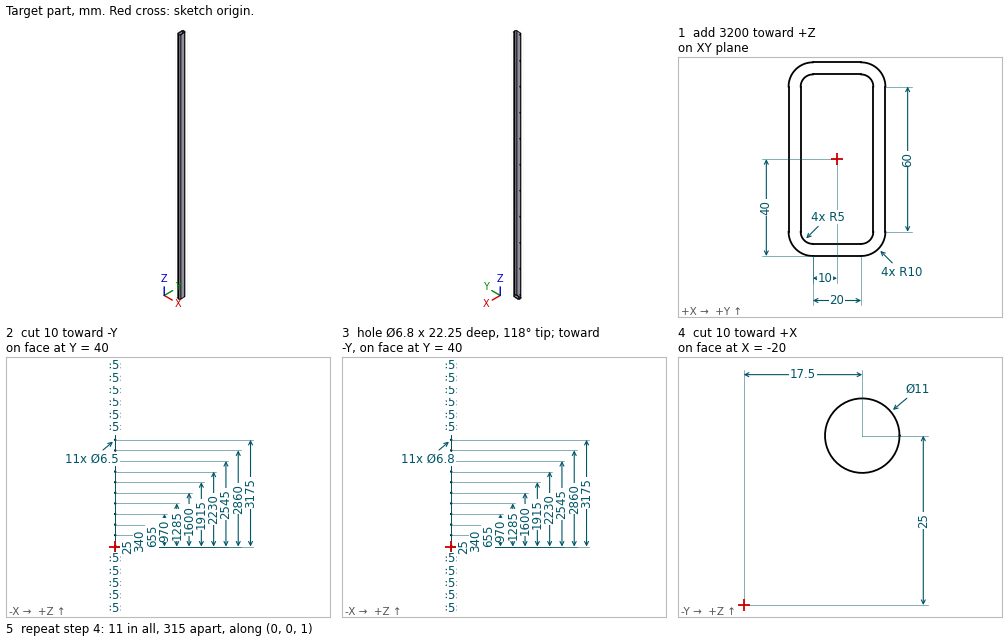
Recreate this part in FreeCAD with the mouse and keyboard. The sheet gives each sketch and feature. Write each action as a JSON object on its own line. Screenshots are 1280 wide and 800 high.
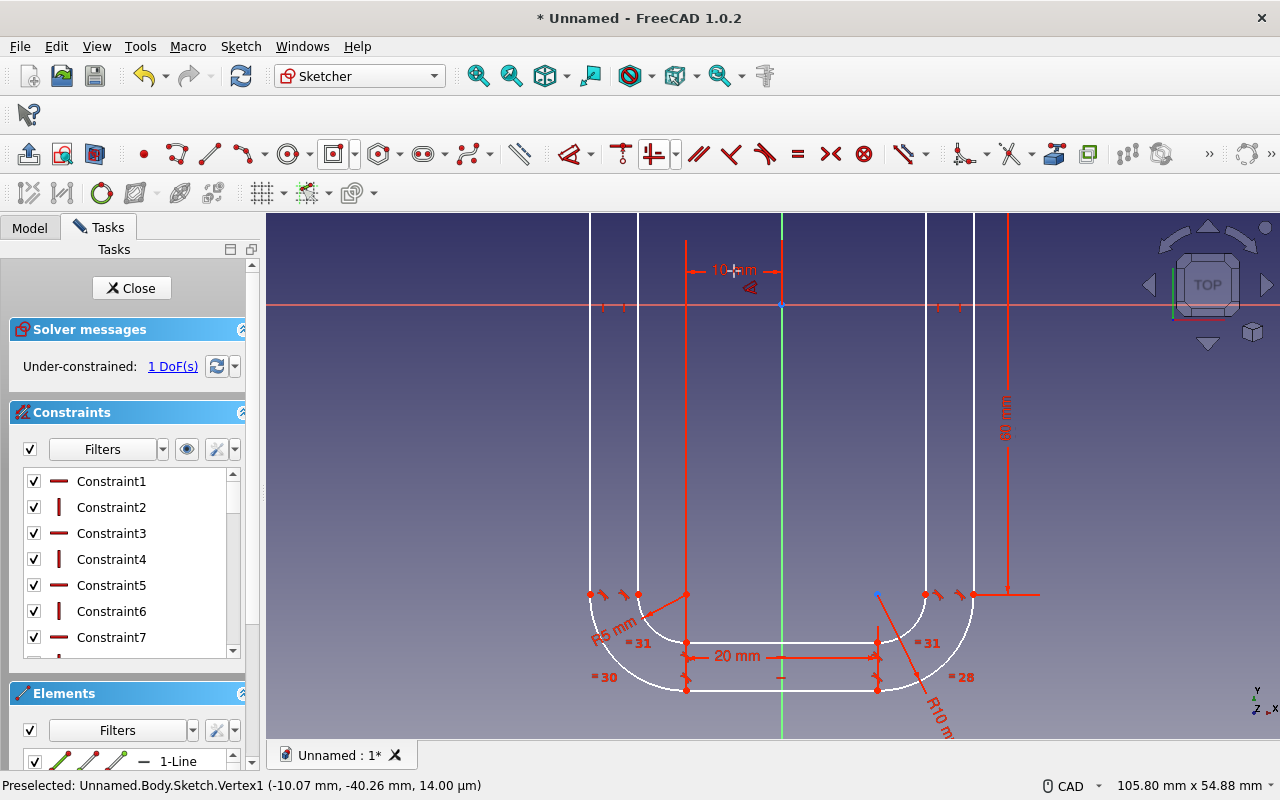
{"action": "left_click", "coordinate": [686, 691]}
{"action": "left_click", "coordinate": [652, 498]}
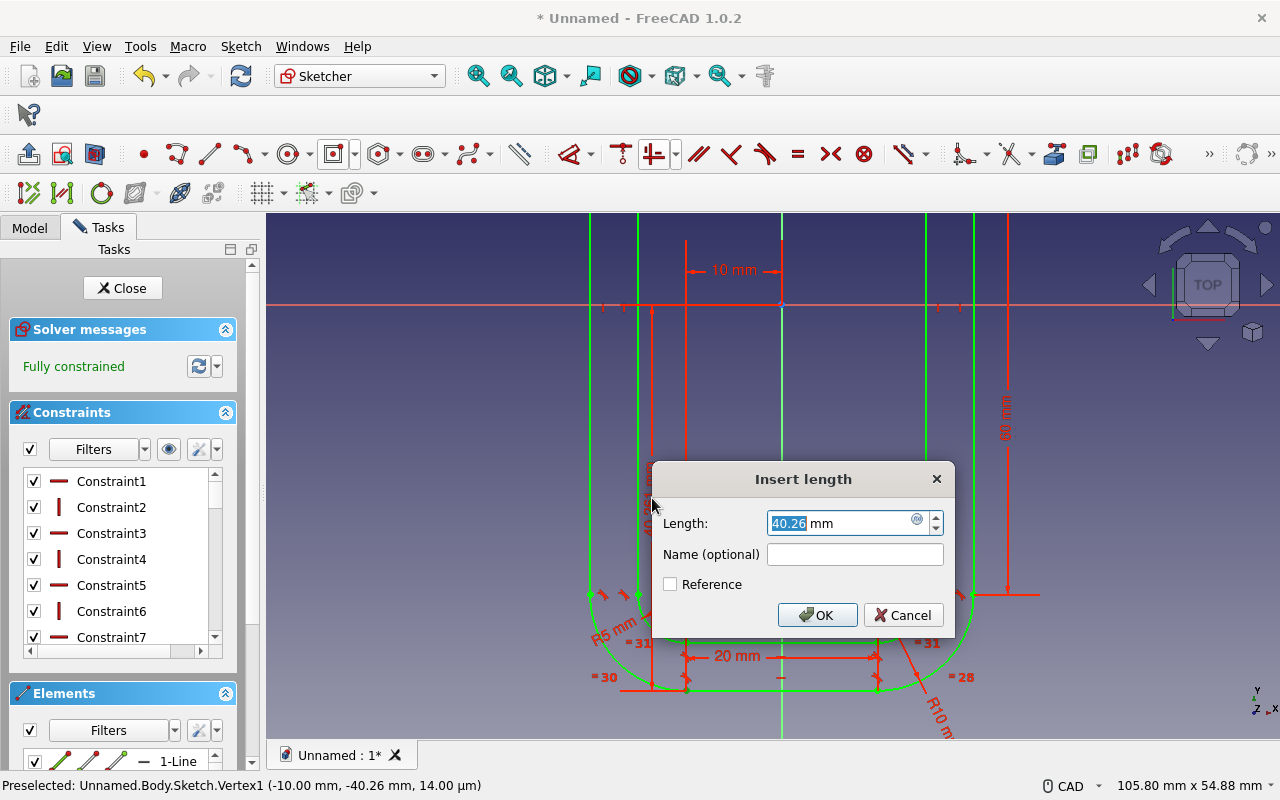
{"action": "type", "text": "40"}
{"action": "key", "text": "Return"}
{"action": "key", "text": "Escape"}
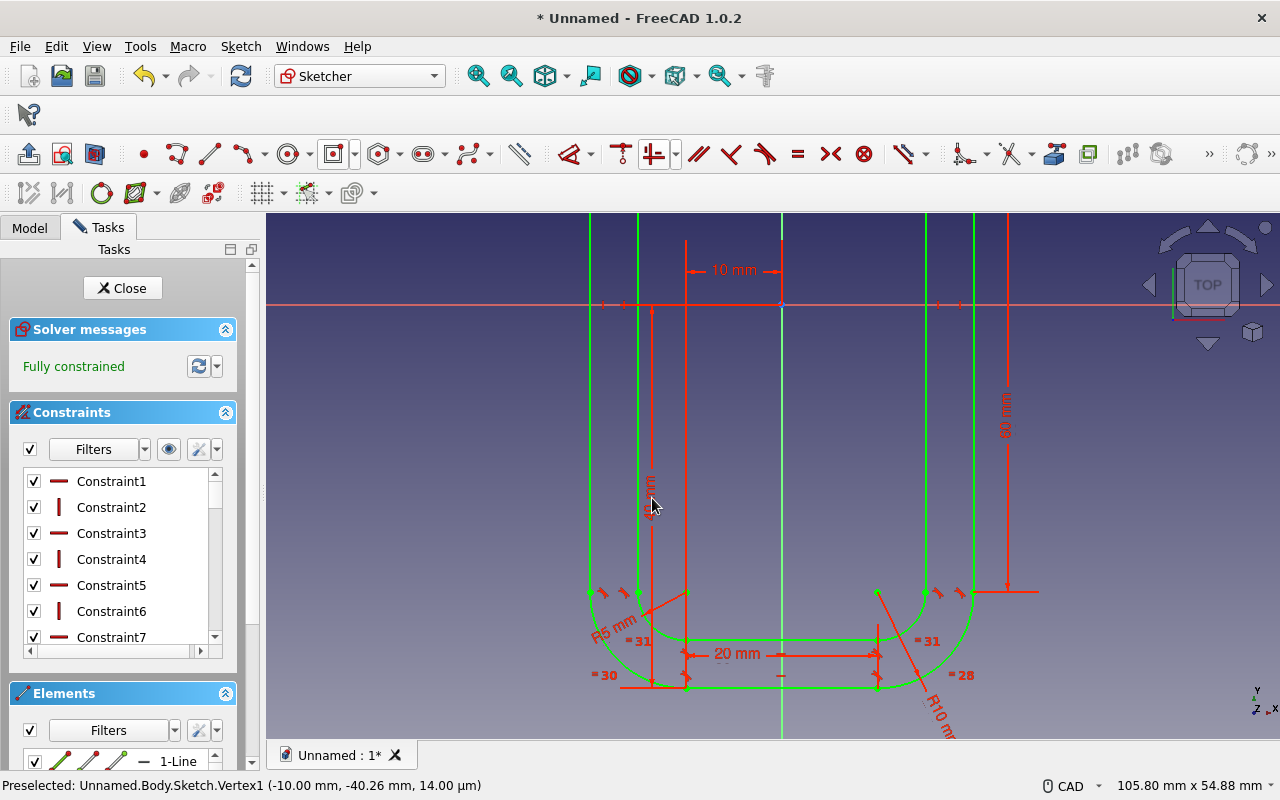
{"action": "left_click", "coordinate": [123, 288]}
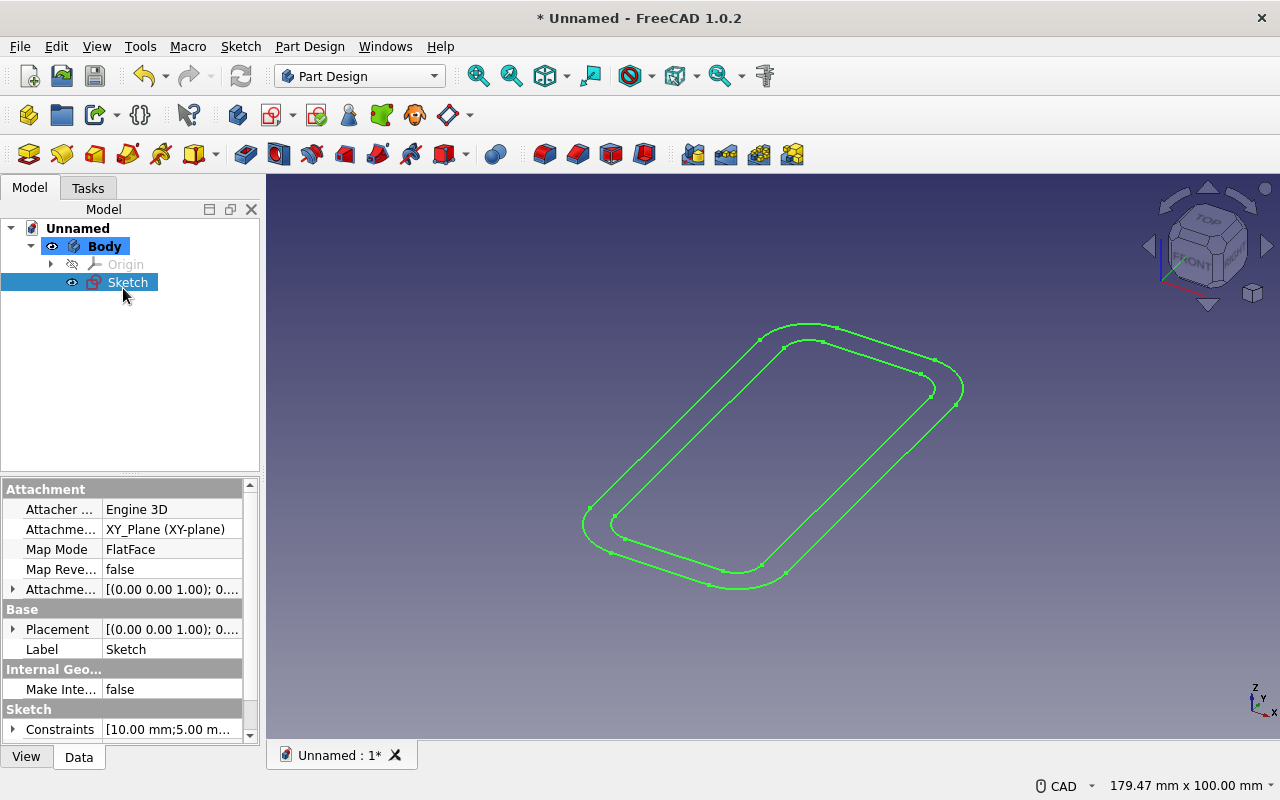
{"action": "left_click", "coordinate": [29, 154]}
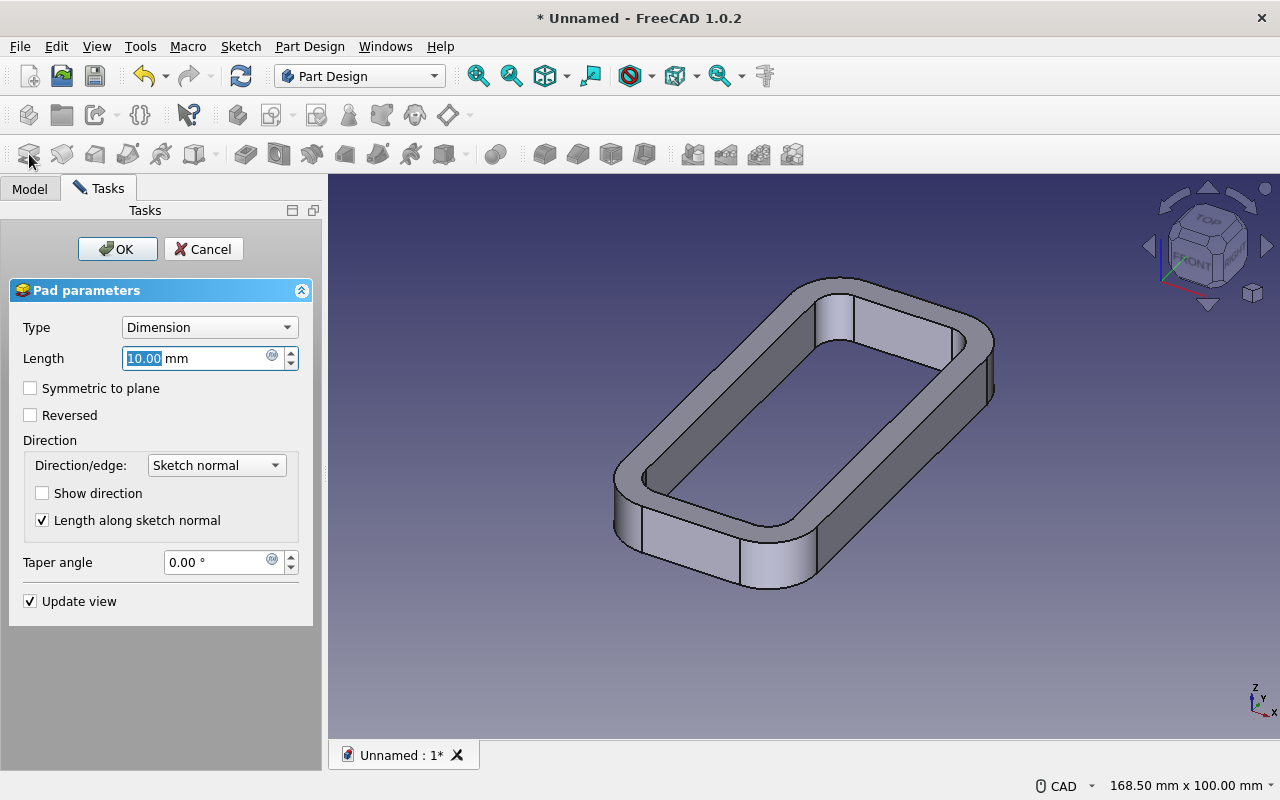
{"action": "type", "text": "3200"}
{"action": "key", "text": "Tab"}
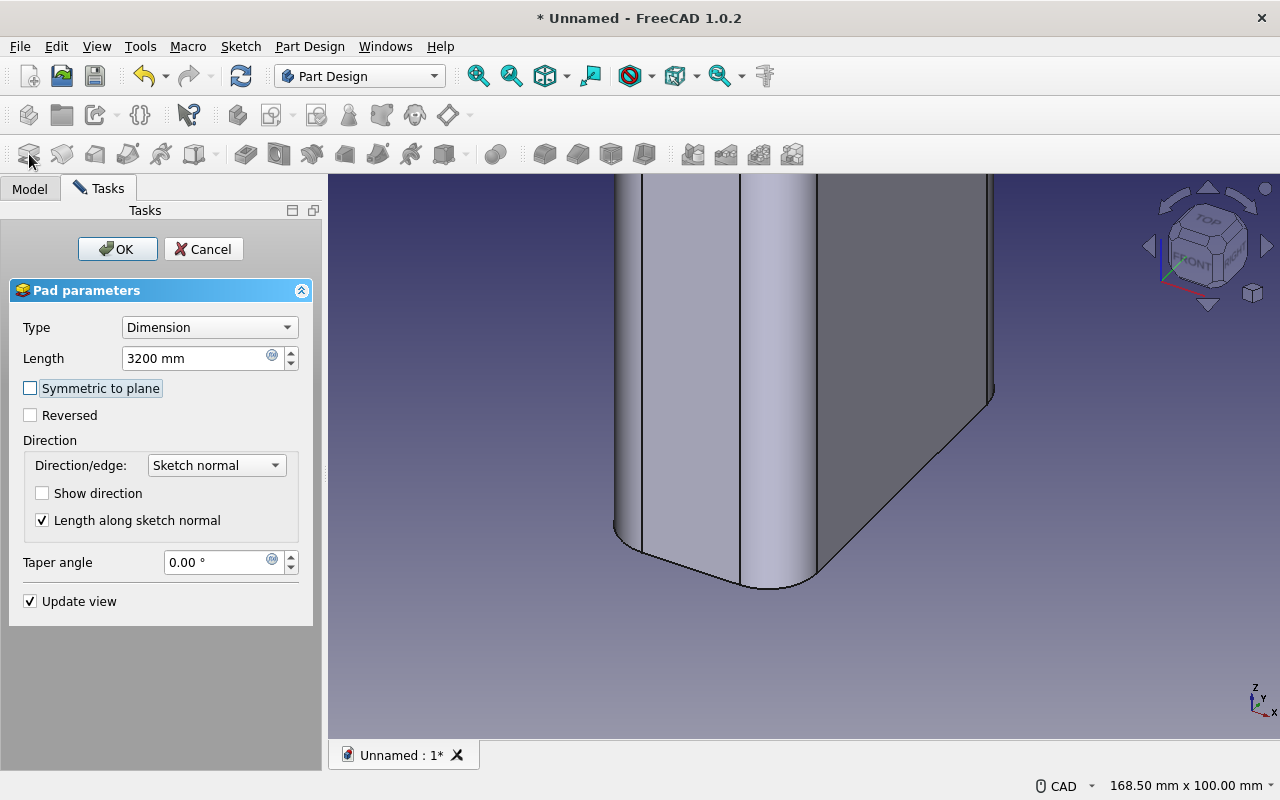
{"action": "left_click", "coordinate": [118, 249]}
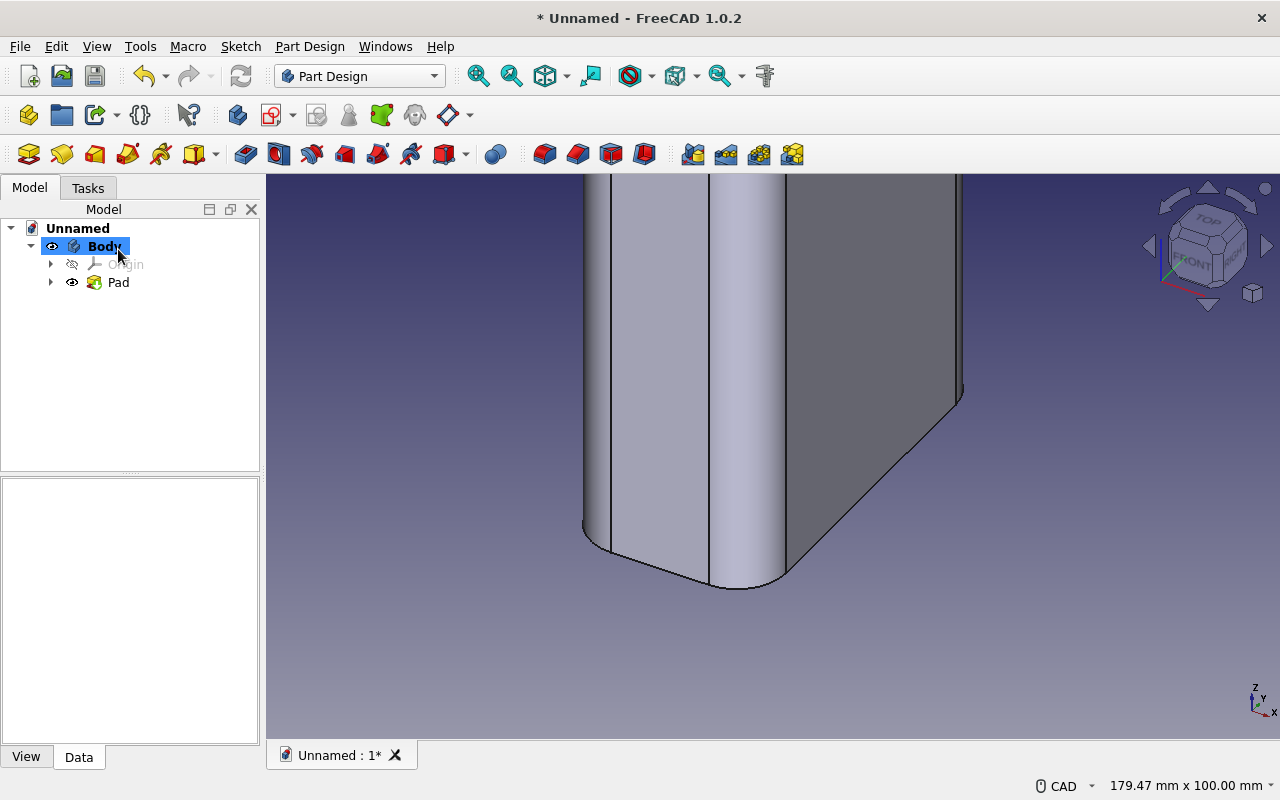
{"action": "key", "text": "v f"}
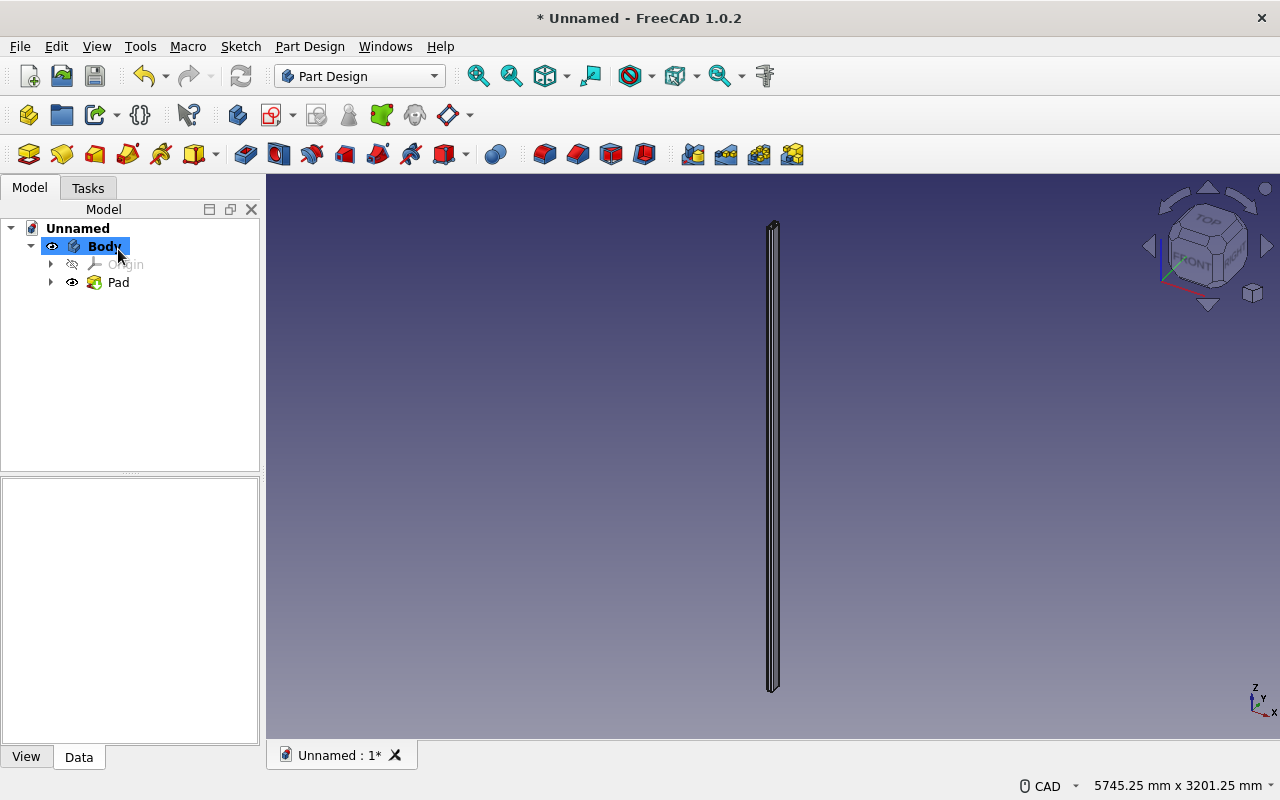
{"action": "key", "text": "4"}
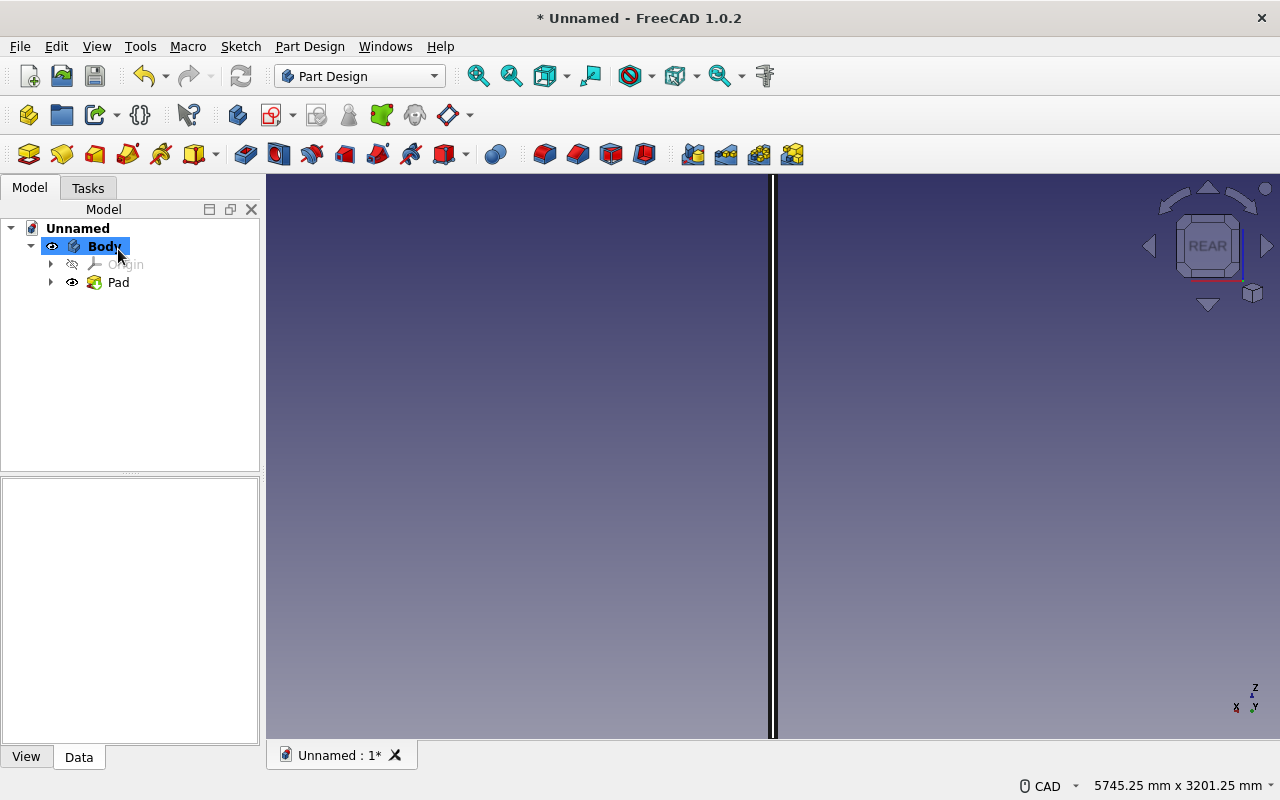
{"action": "left_click", "coordinate": [479, 76]}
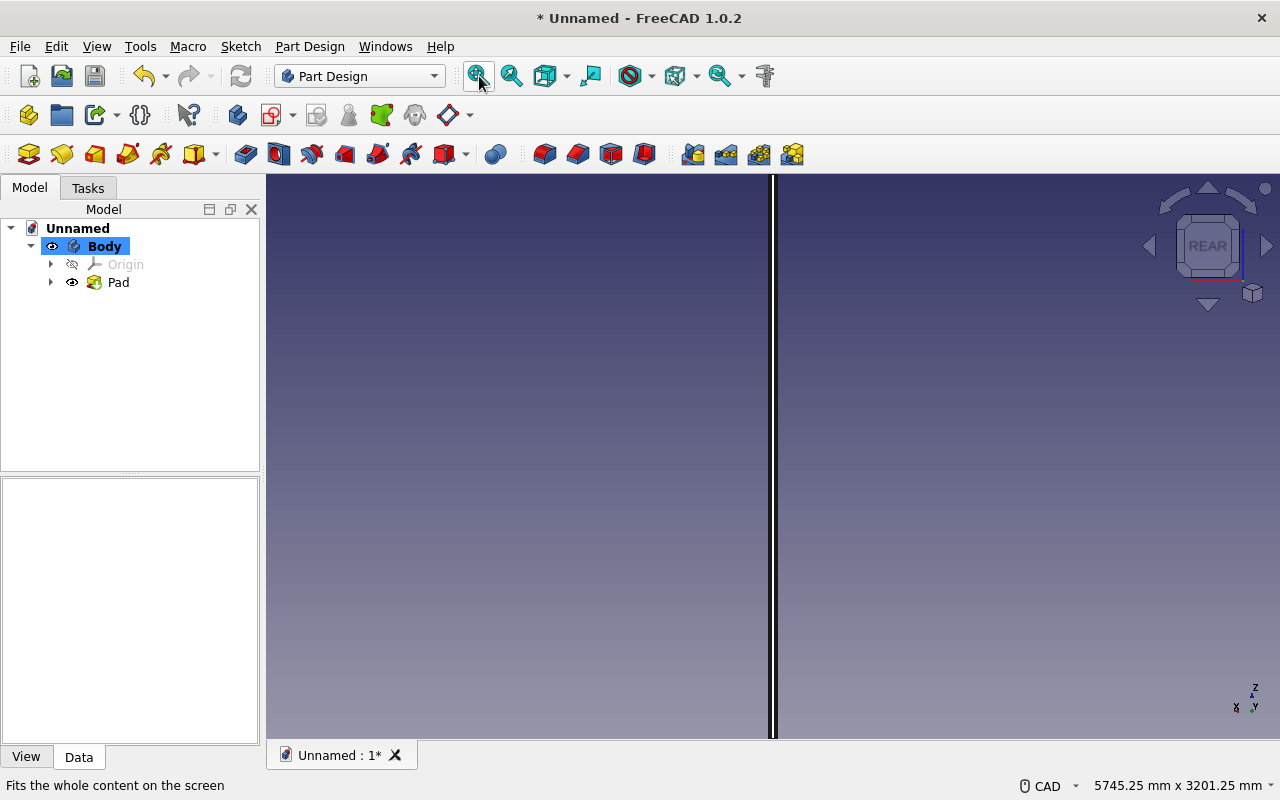
{"action": "scroll", "coordinate": [773, 213], "scroll_direction": "up", "scroll_amount": 10}